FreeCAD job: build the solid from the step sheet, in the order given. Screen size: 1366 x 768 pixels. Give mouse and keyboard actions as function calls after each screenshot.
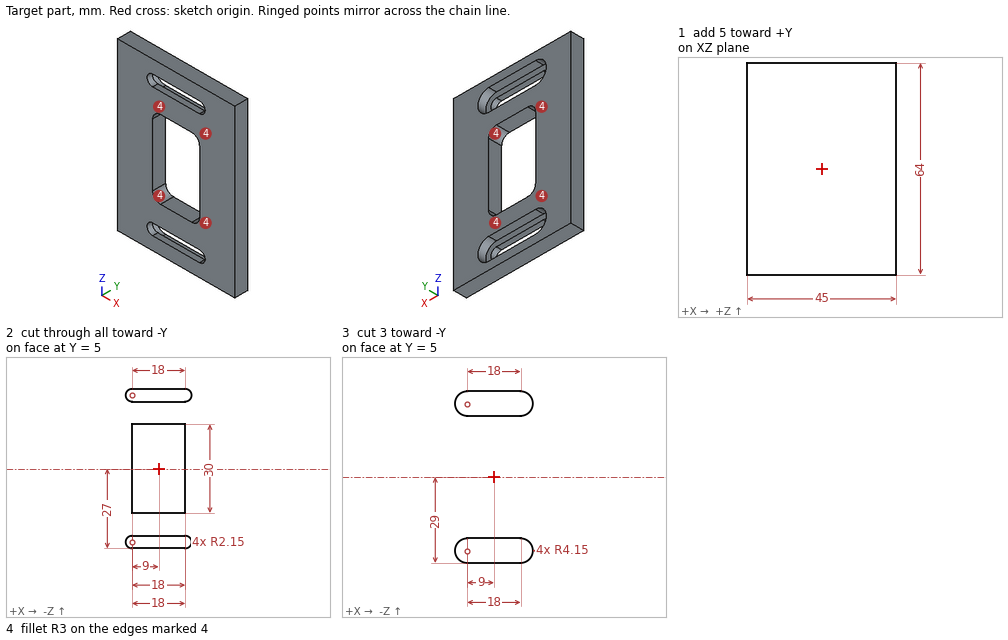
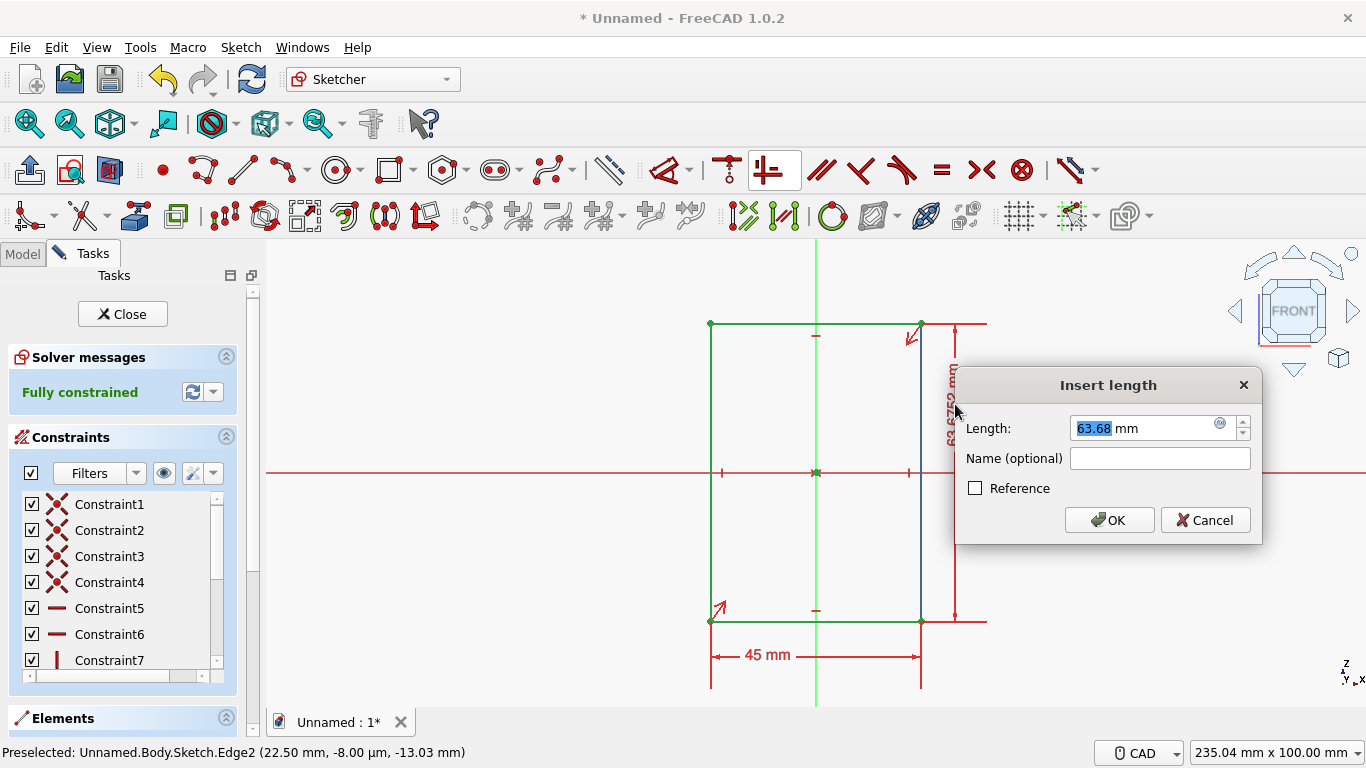
text(64)
key(Return)
key(Escape)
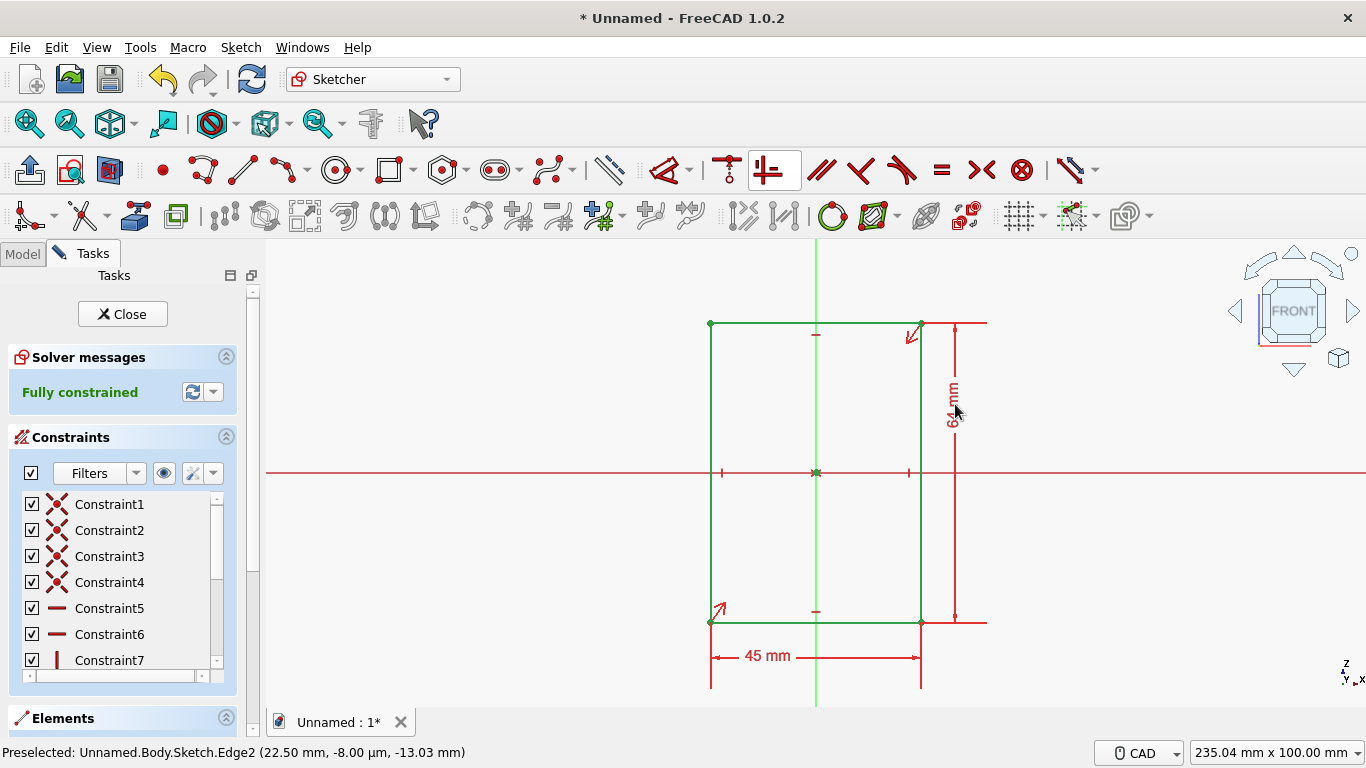
click(123, 314)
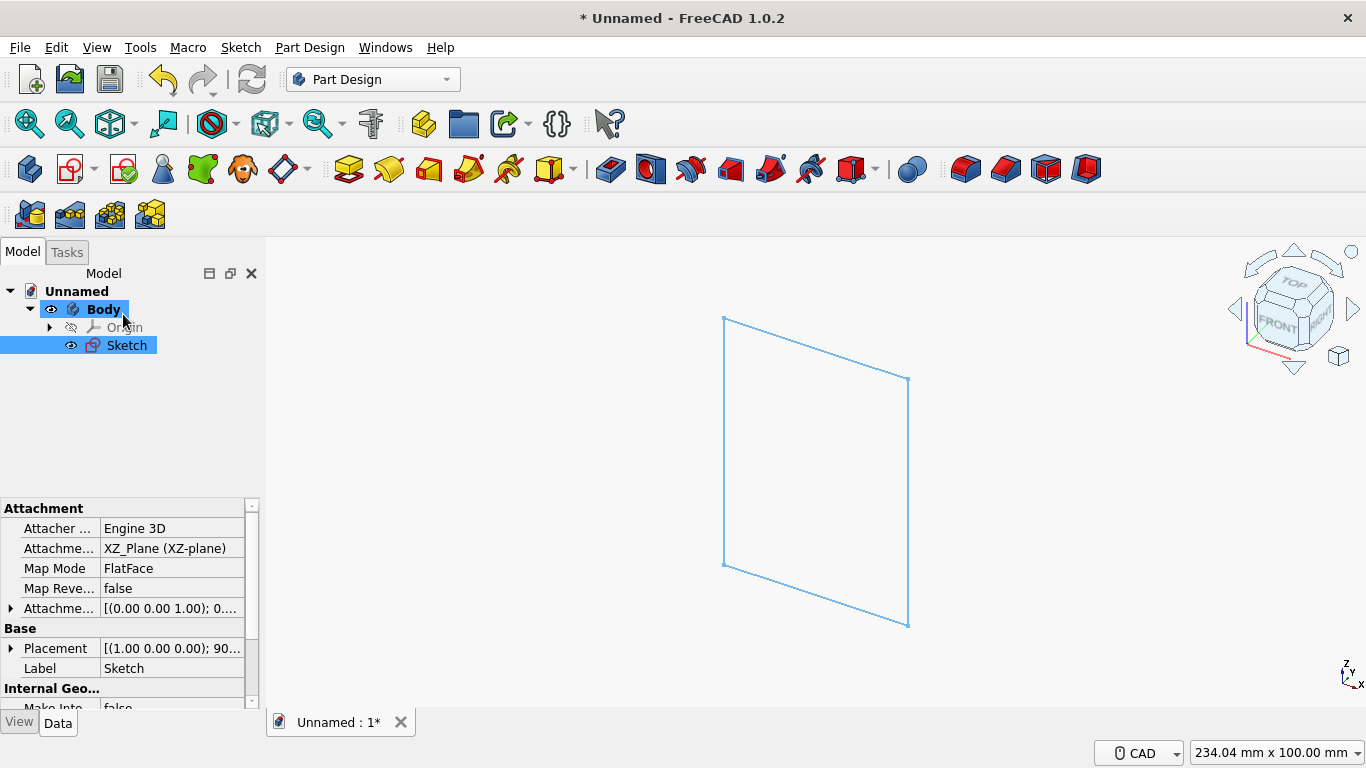
click(350, 170)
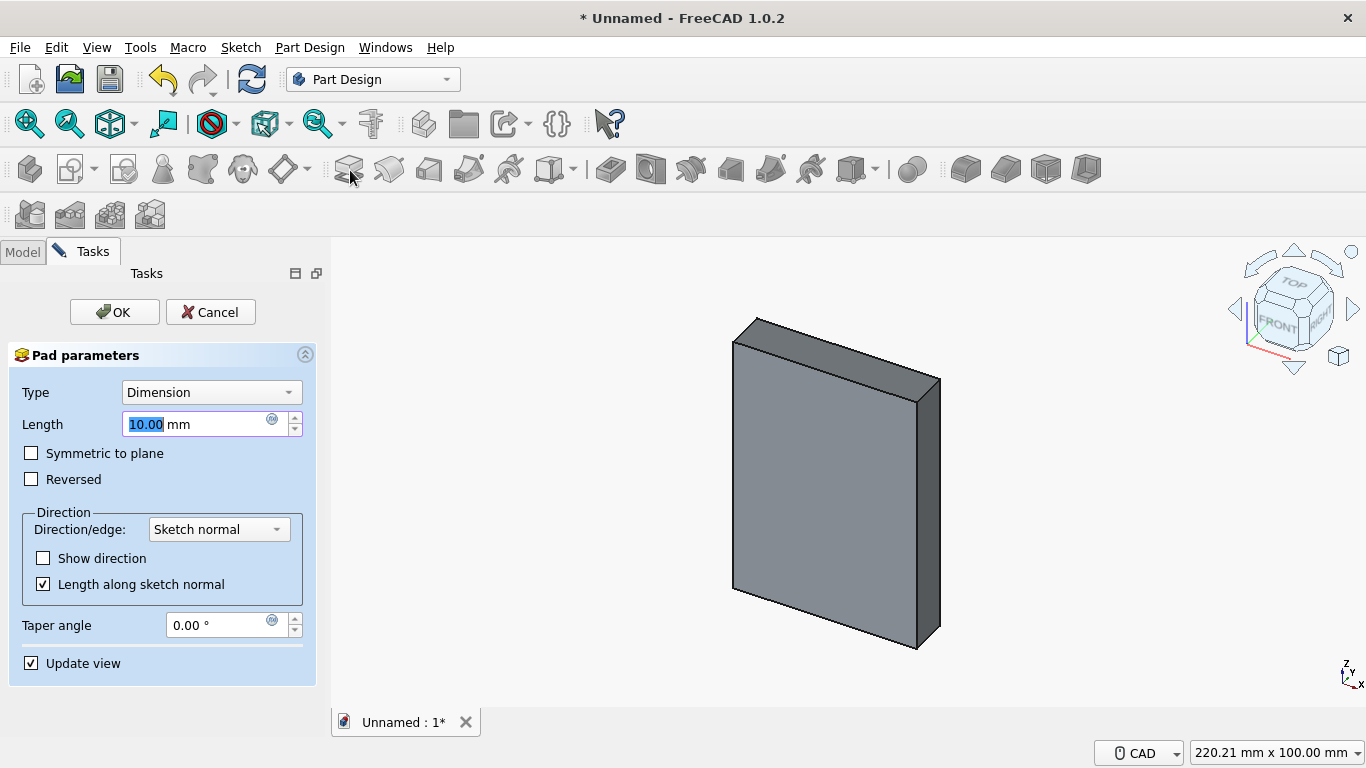
text(5)
key(Tab)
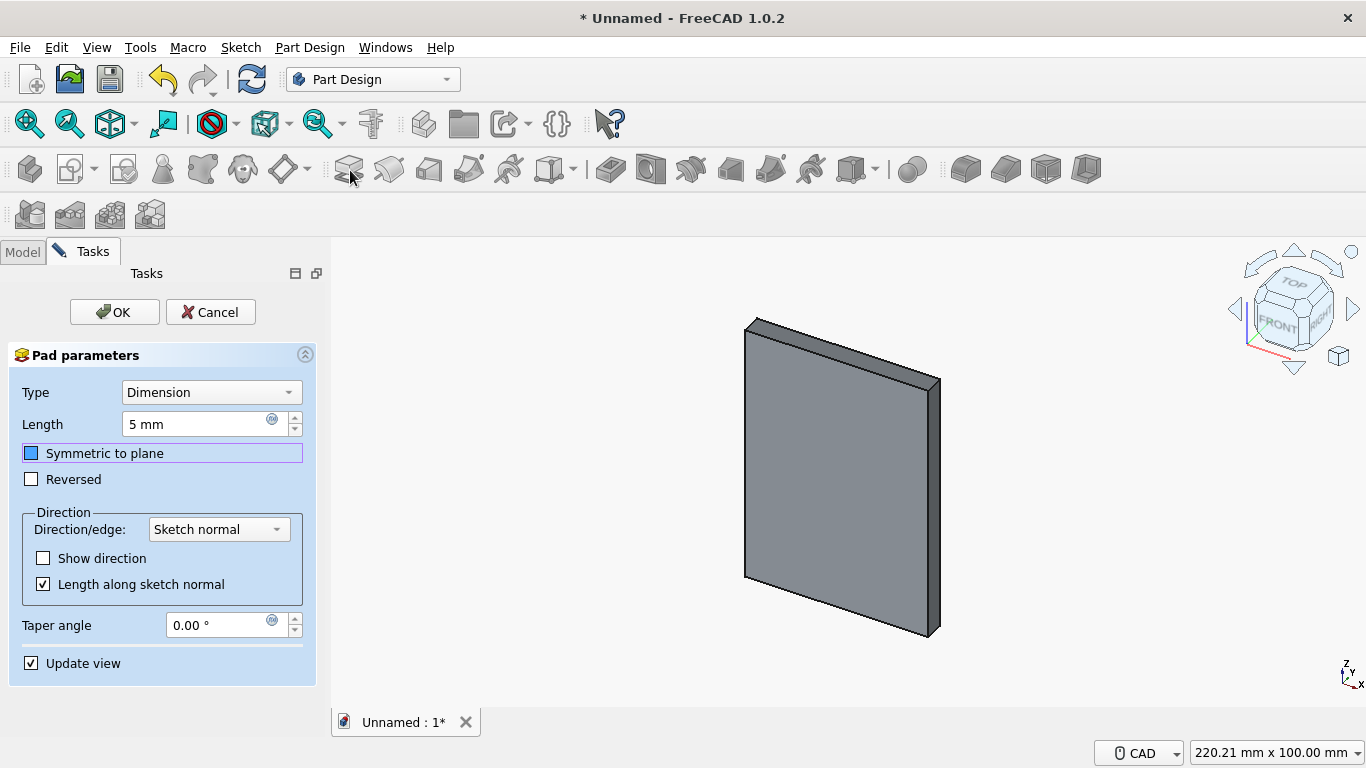
click(30, 479)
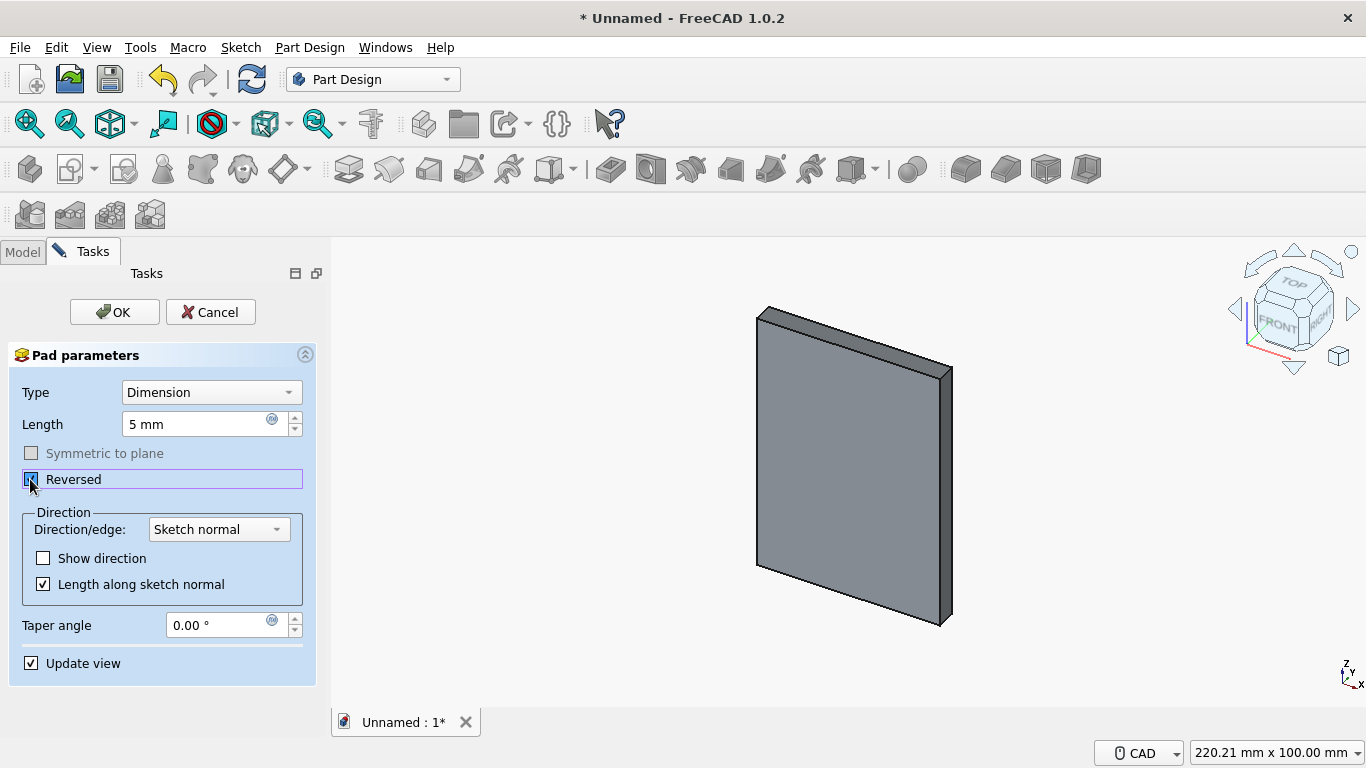
click(115, 312)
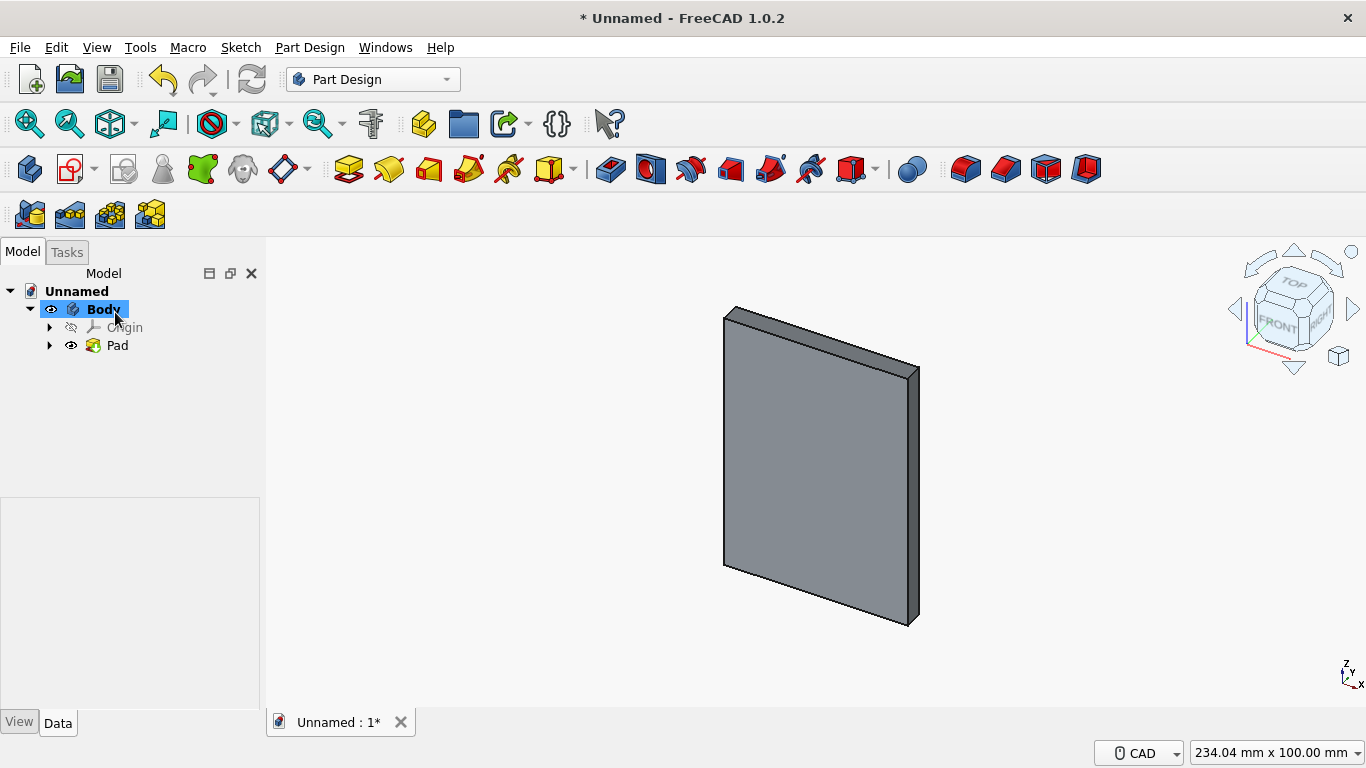
key(4)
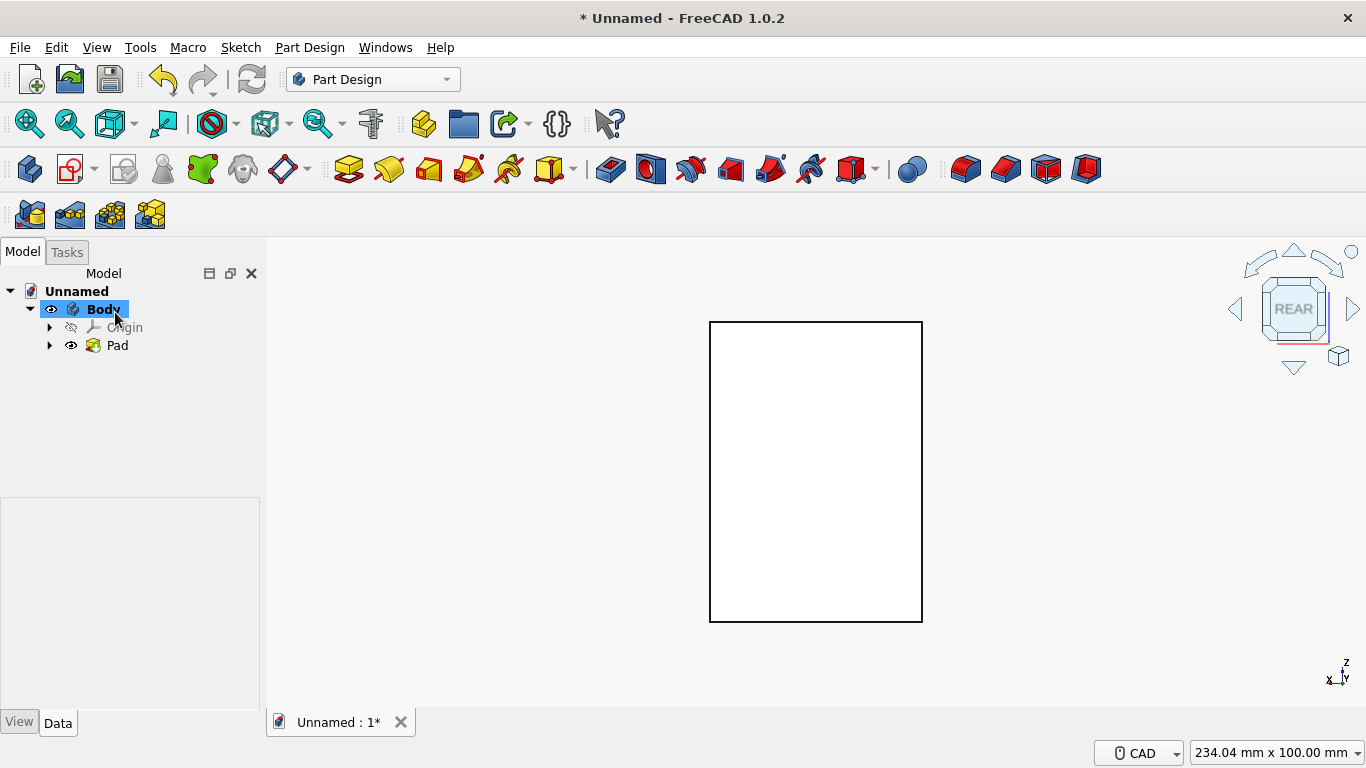
click(816, 428)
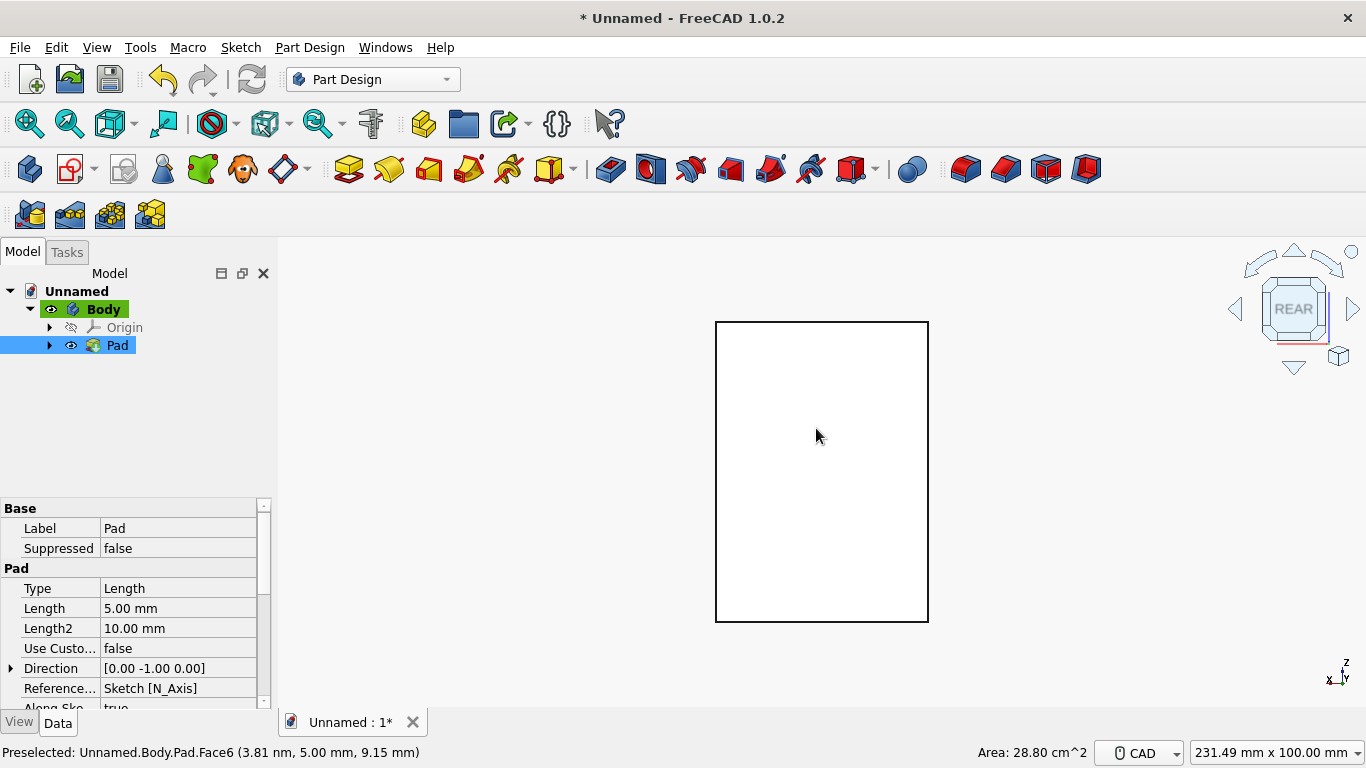
click(70, 170)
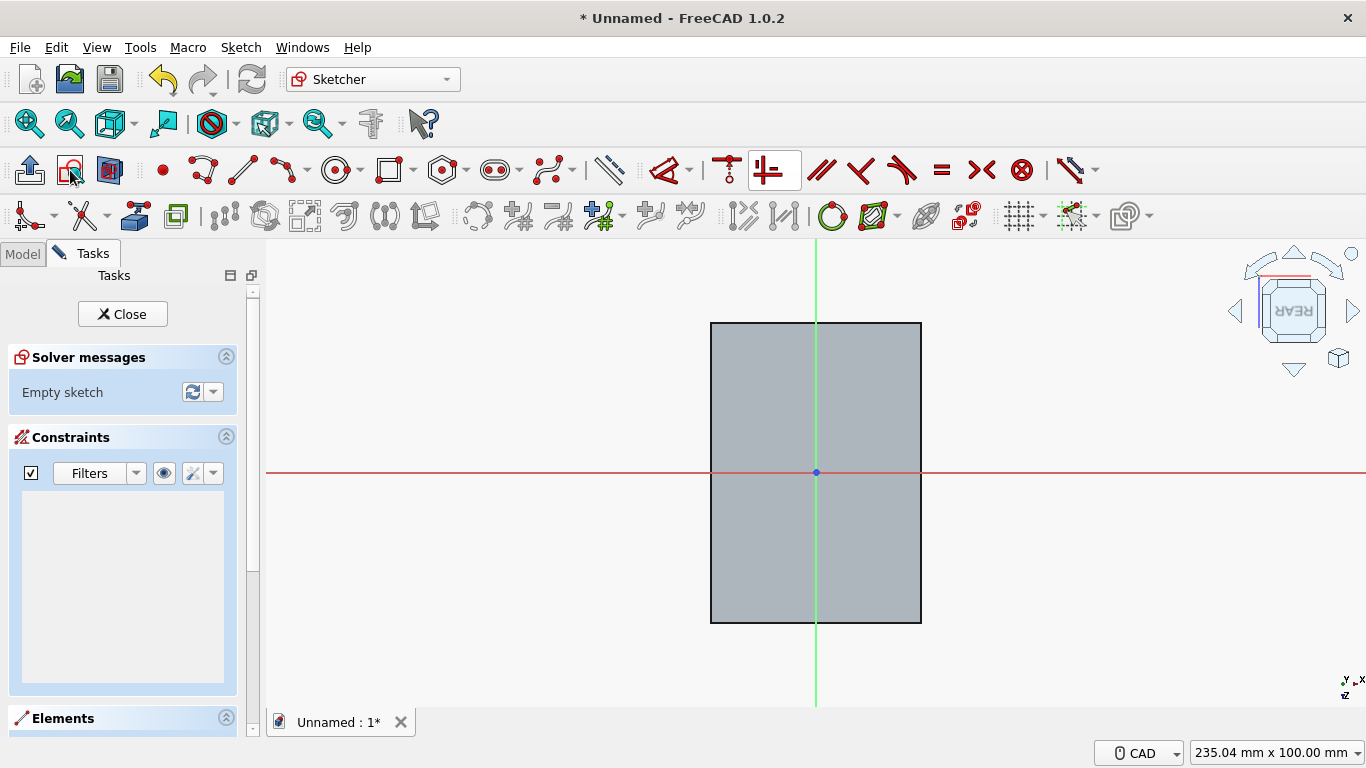
key(g)
key(v)